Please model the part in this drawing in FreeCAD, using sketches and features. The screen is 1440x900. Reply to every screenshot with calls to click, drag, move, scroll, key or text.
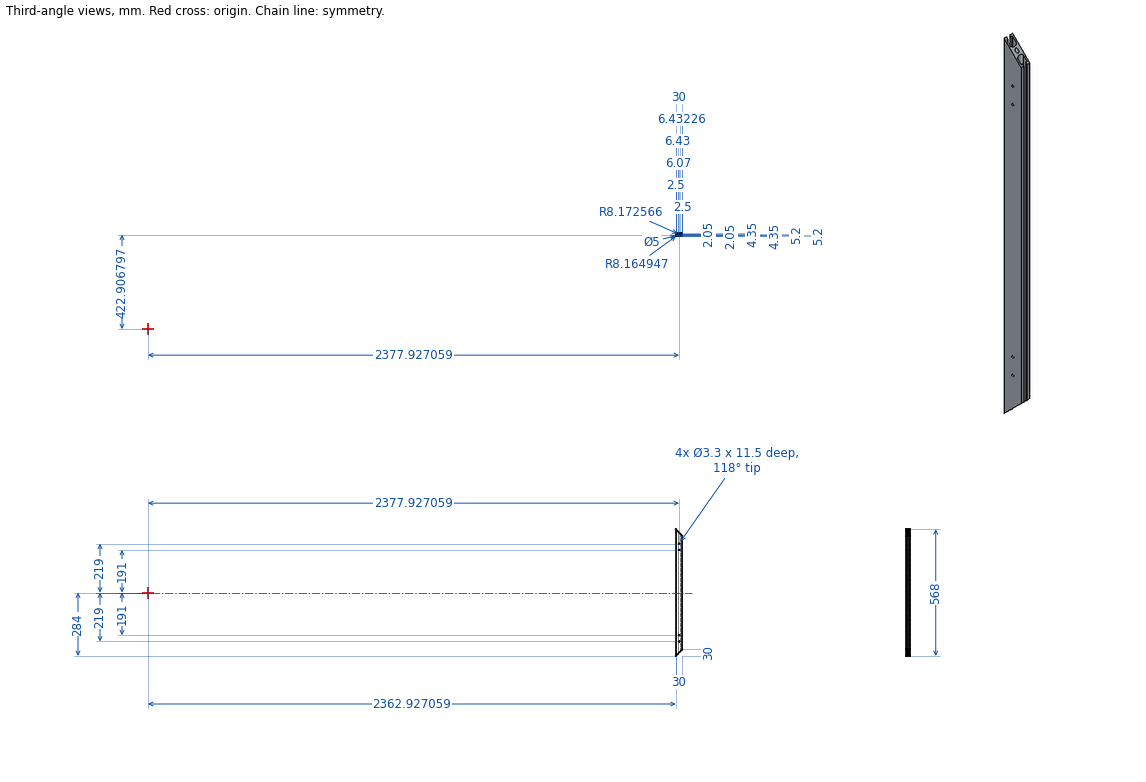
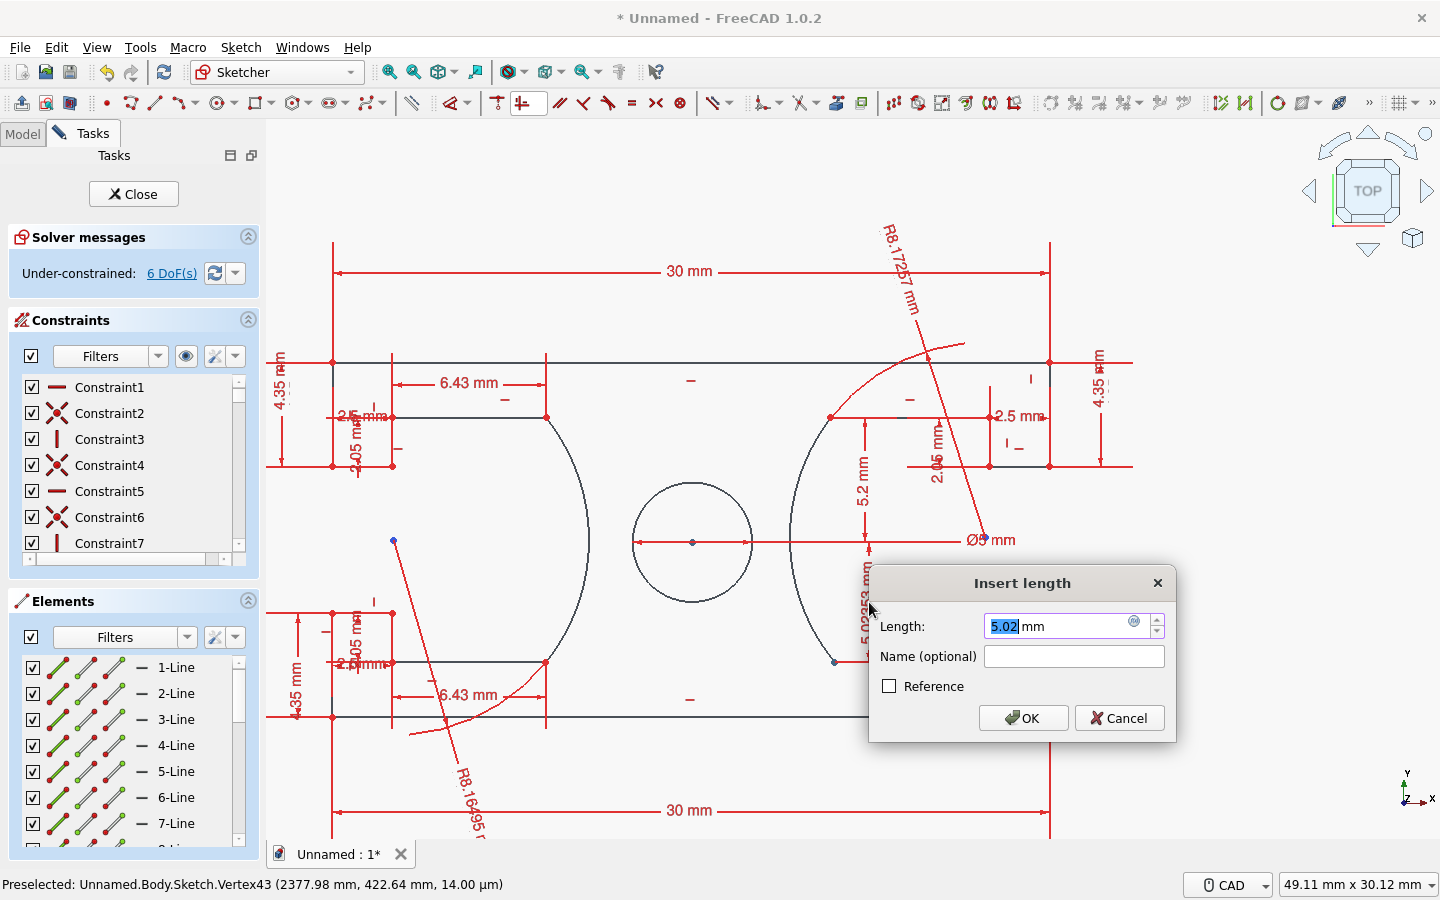
text(5.2)
key(Return)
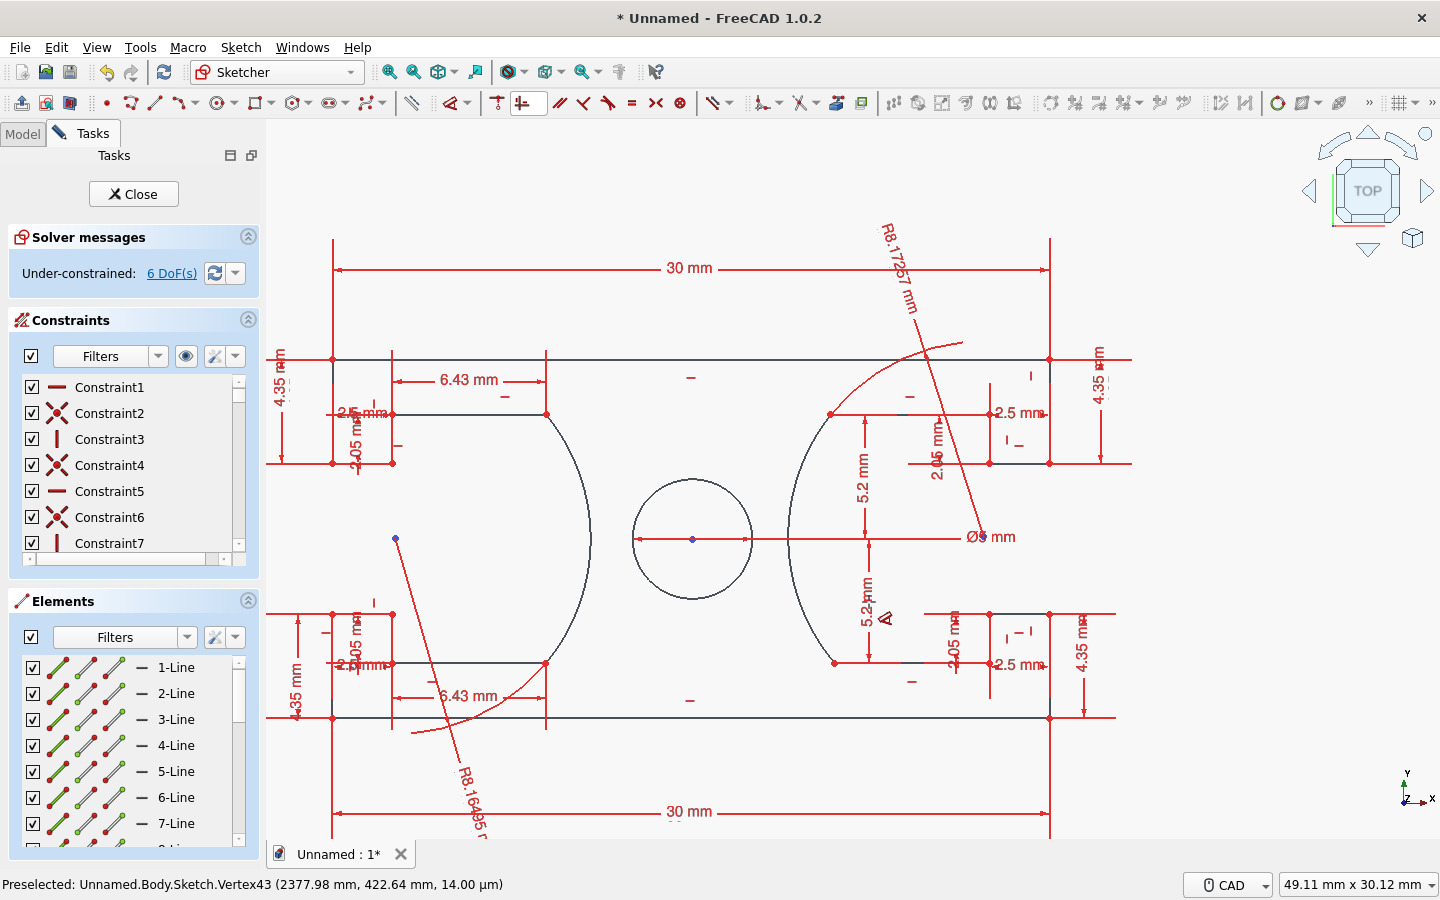
click(546, 415)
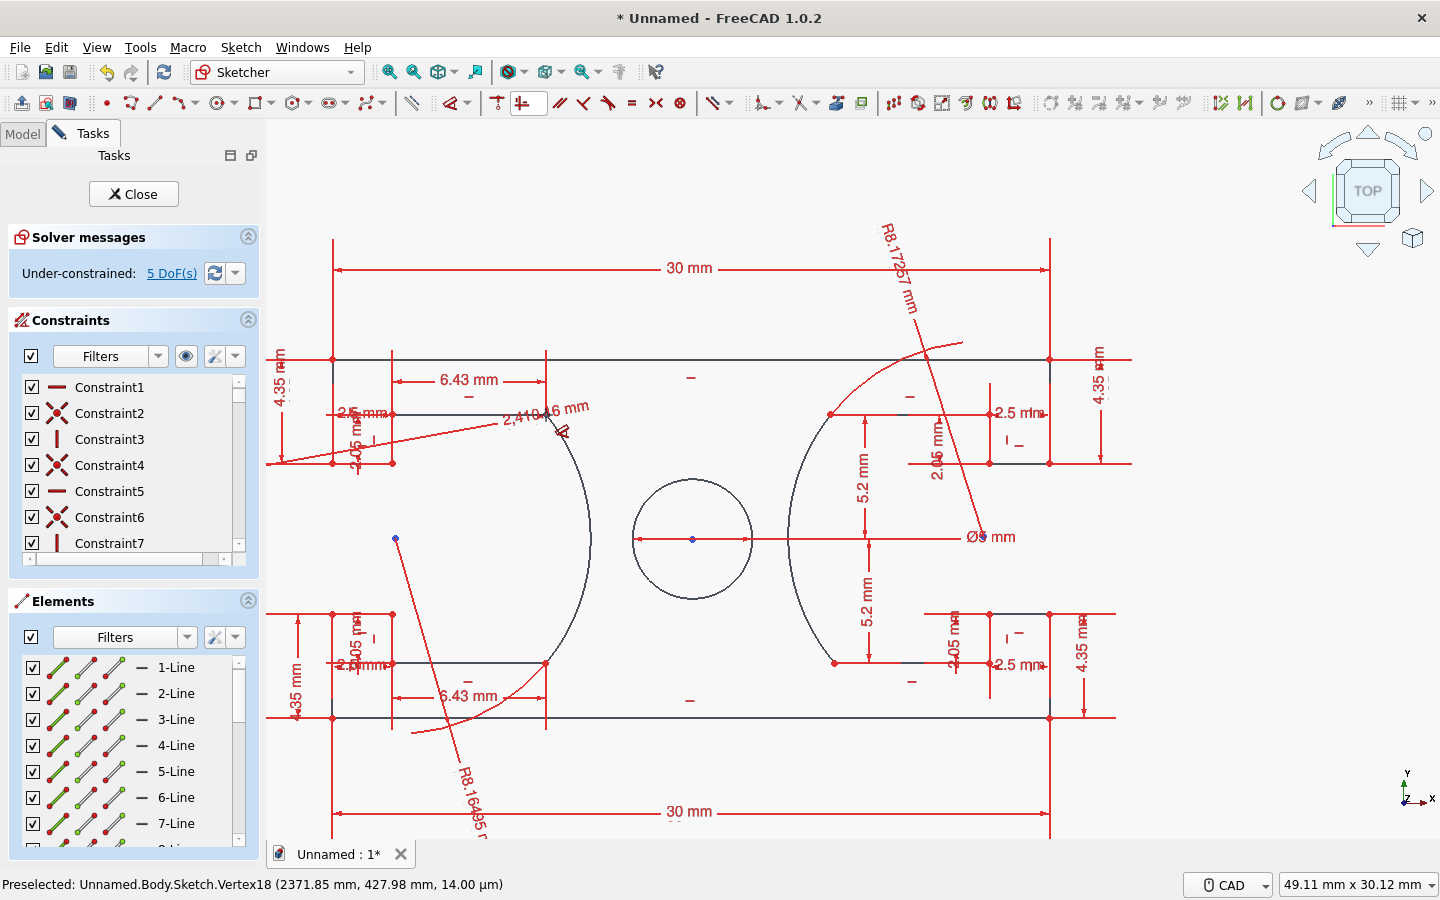
click(692, 539)
click(619, 381)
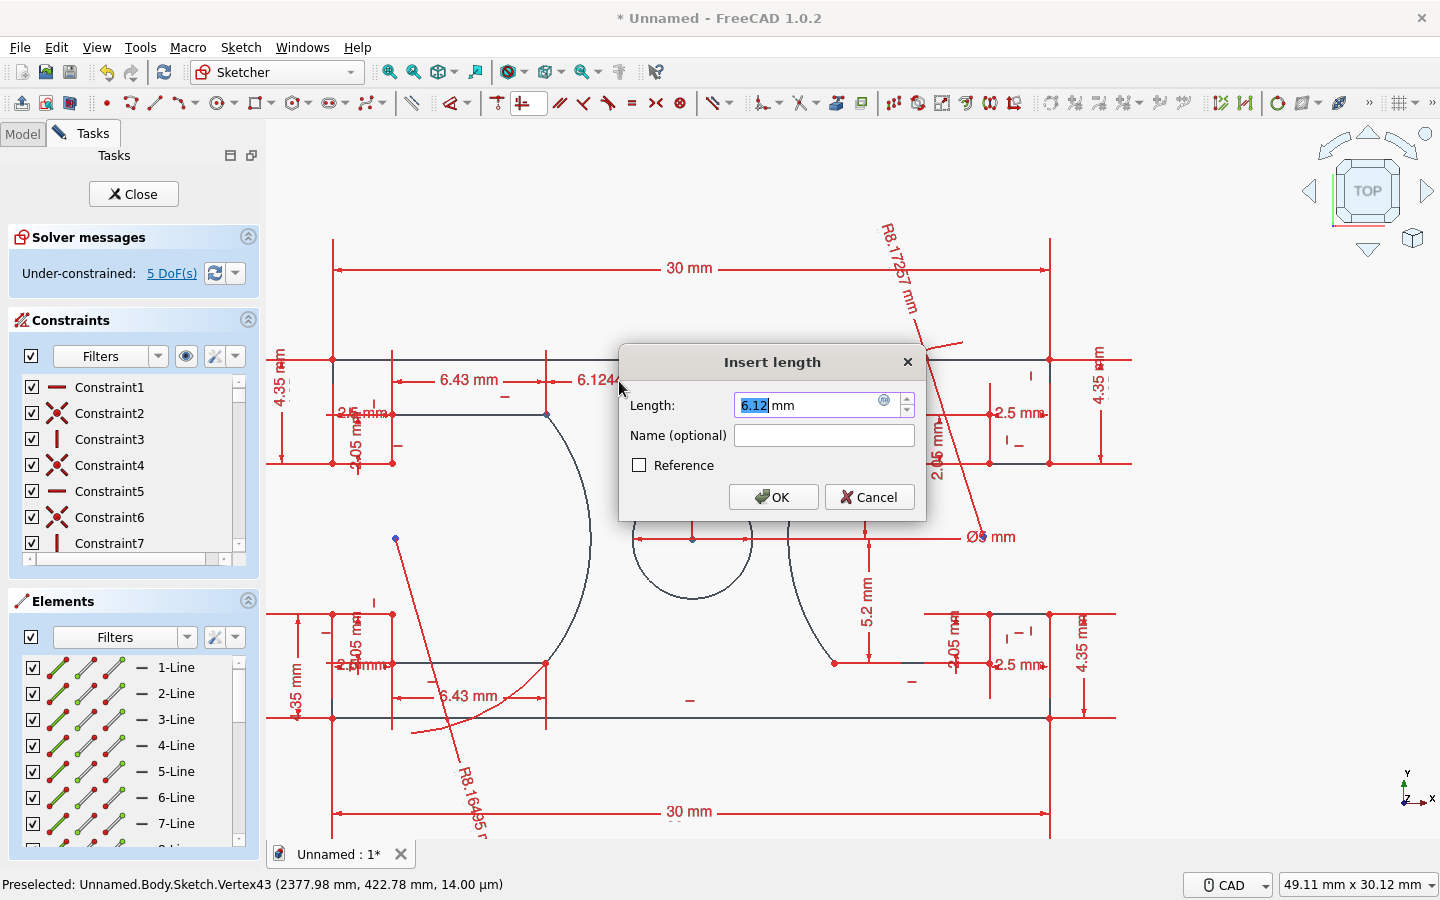
text(6.07)
key(Return)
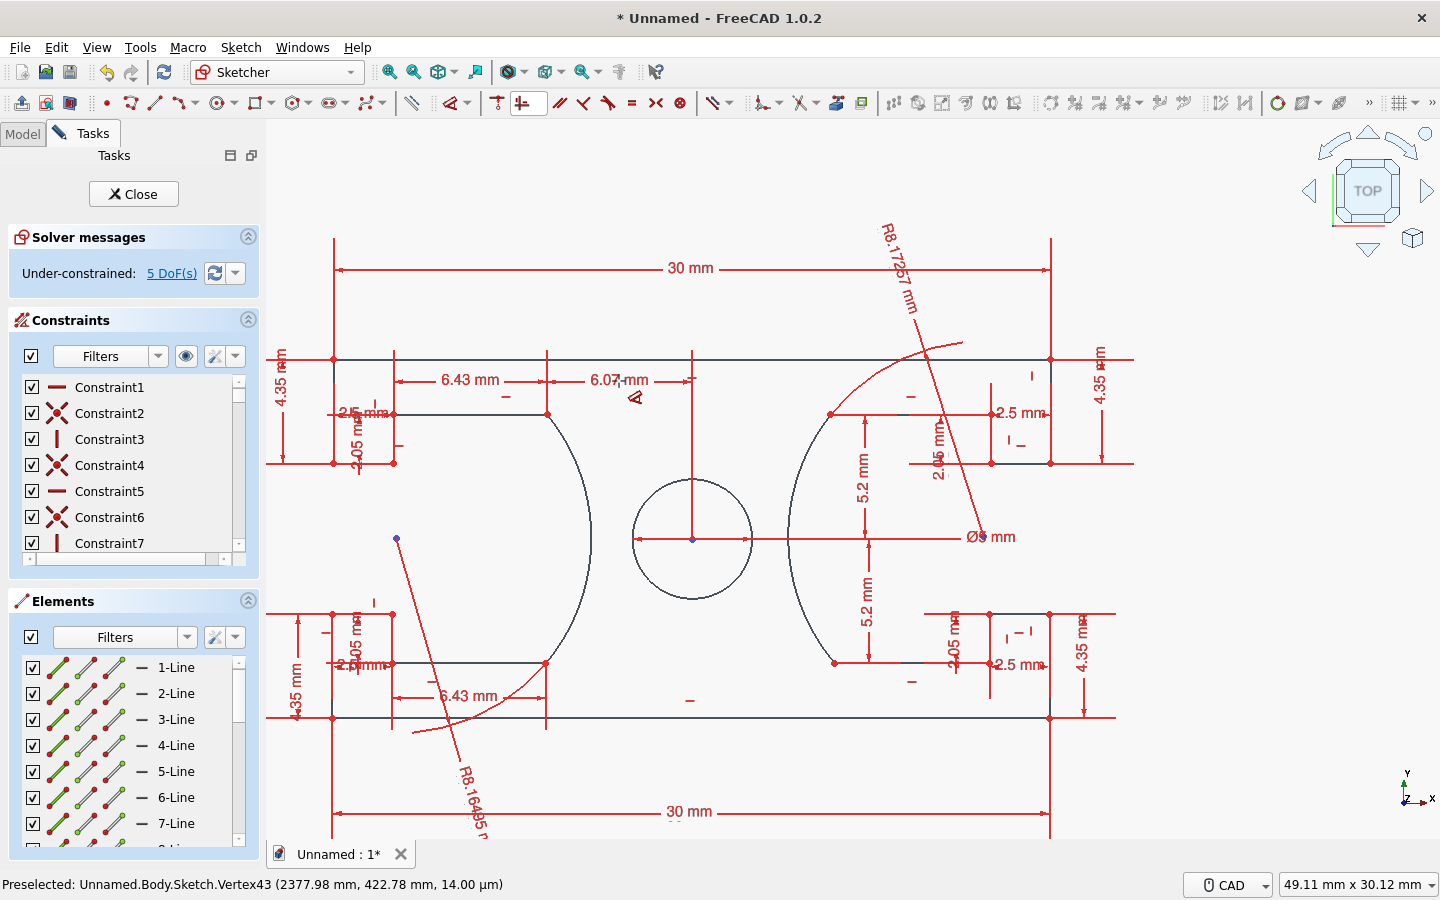
click(546, 663)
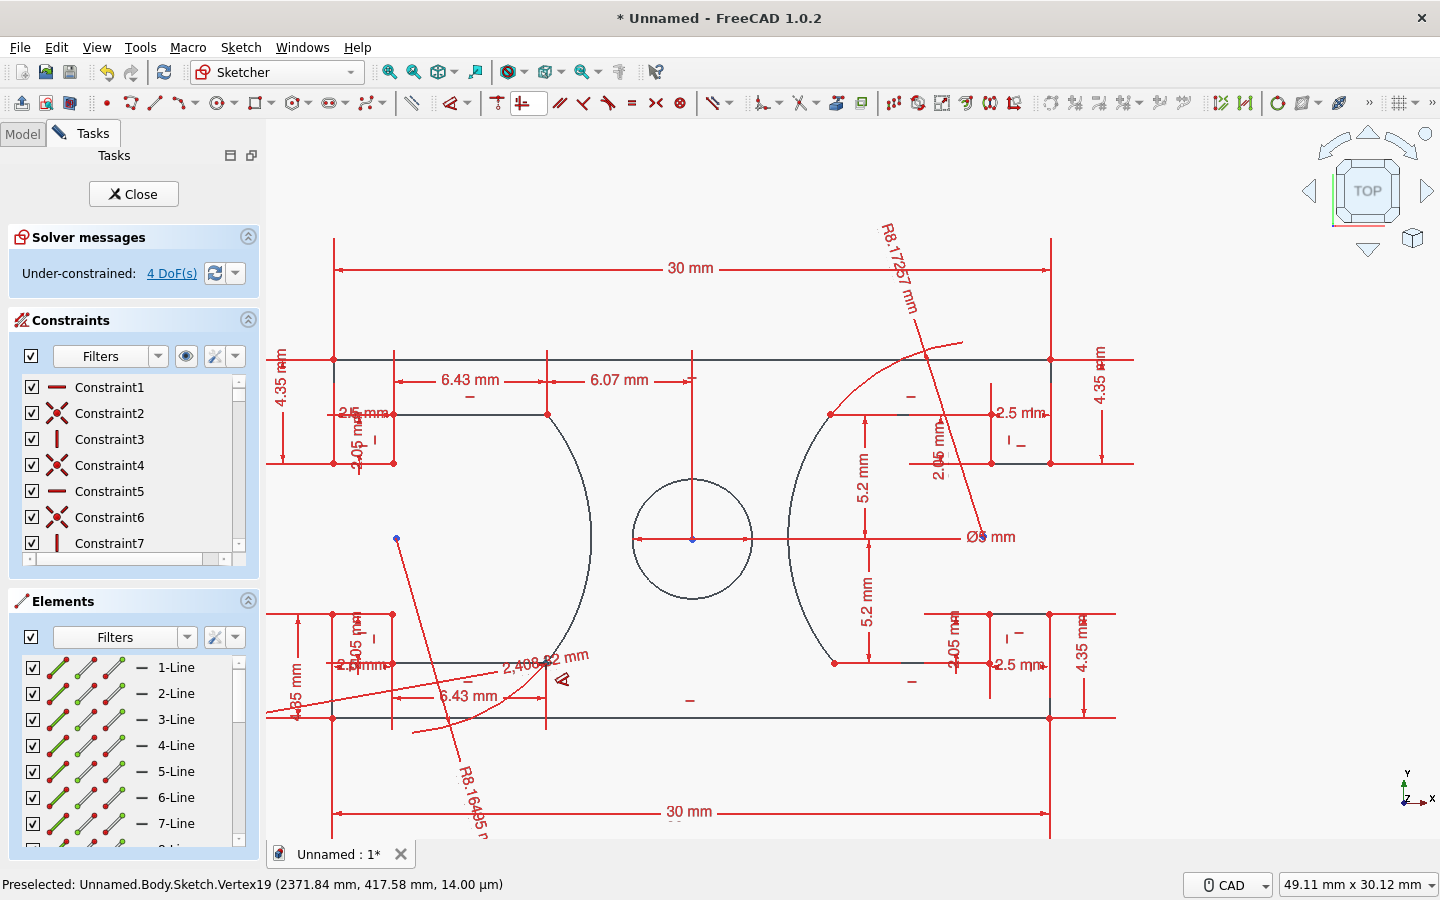
click(692, 539)
click(619, 697)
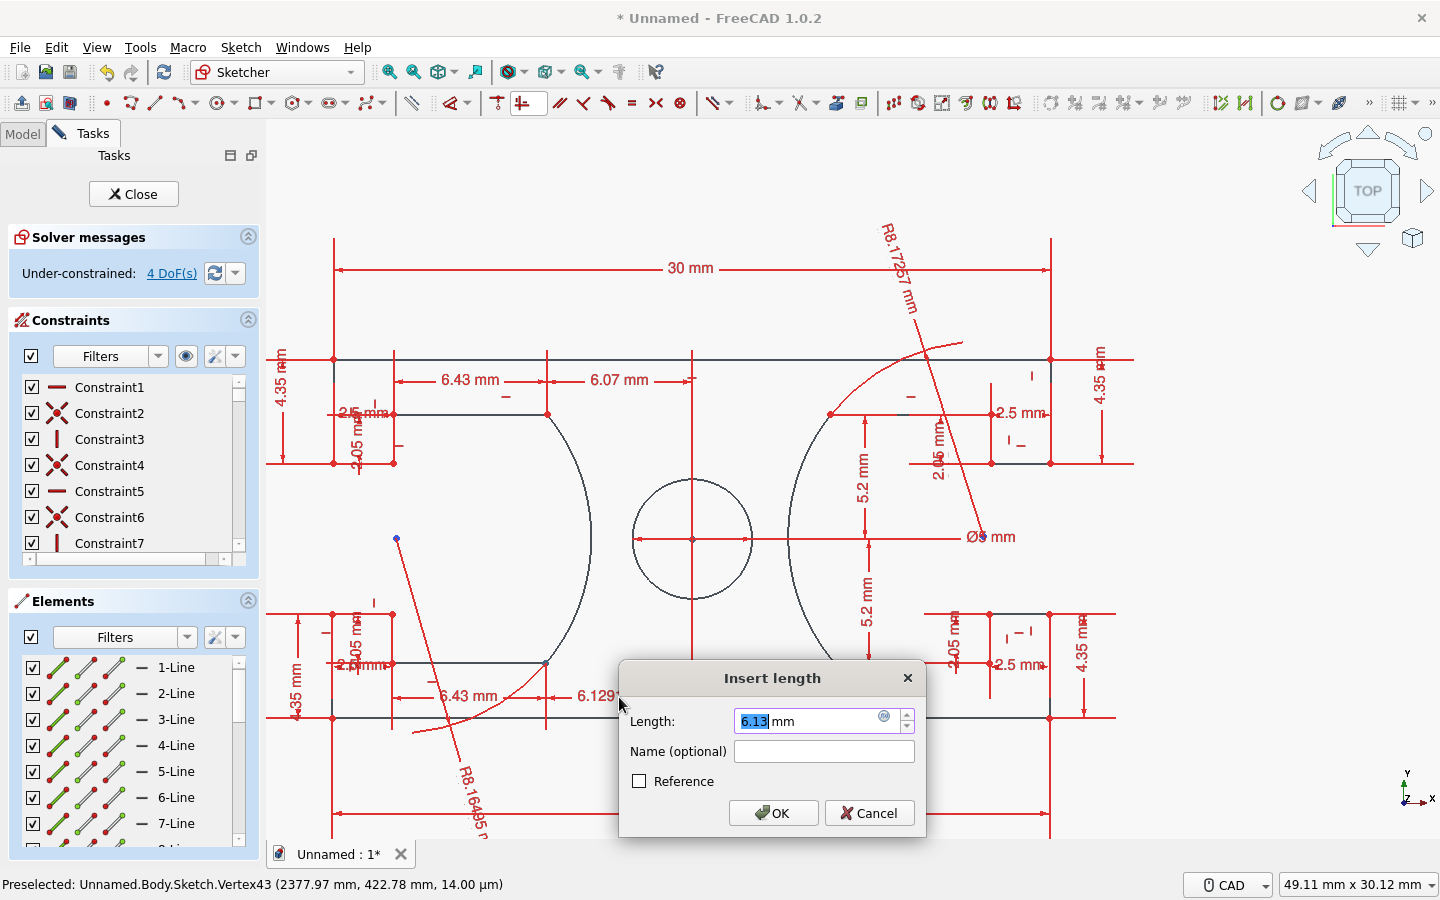
text(6.07)
key(Return)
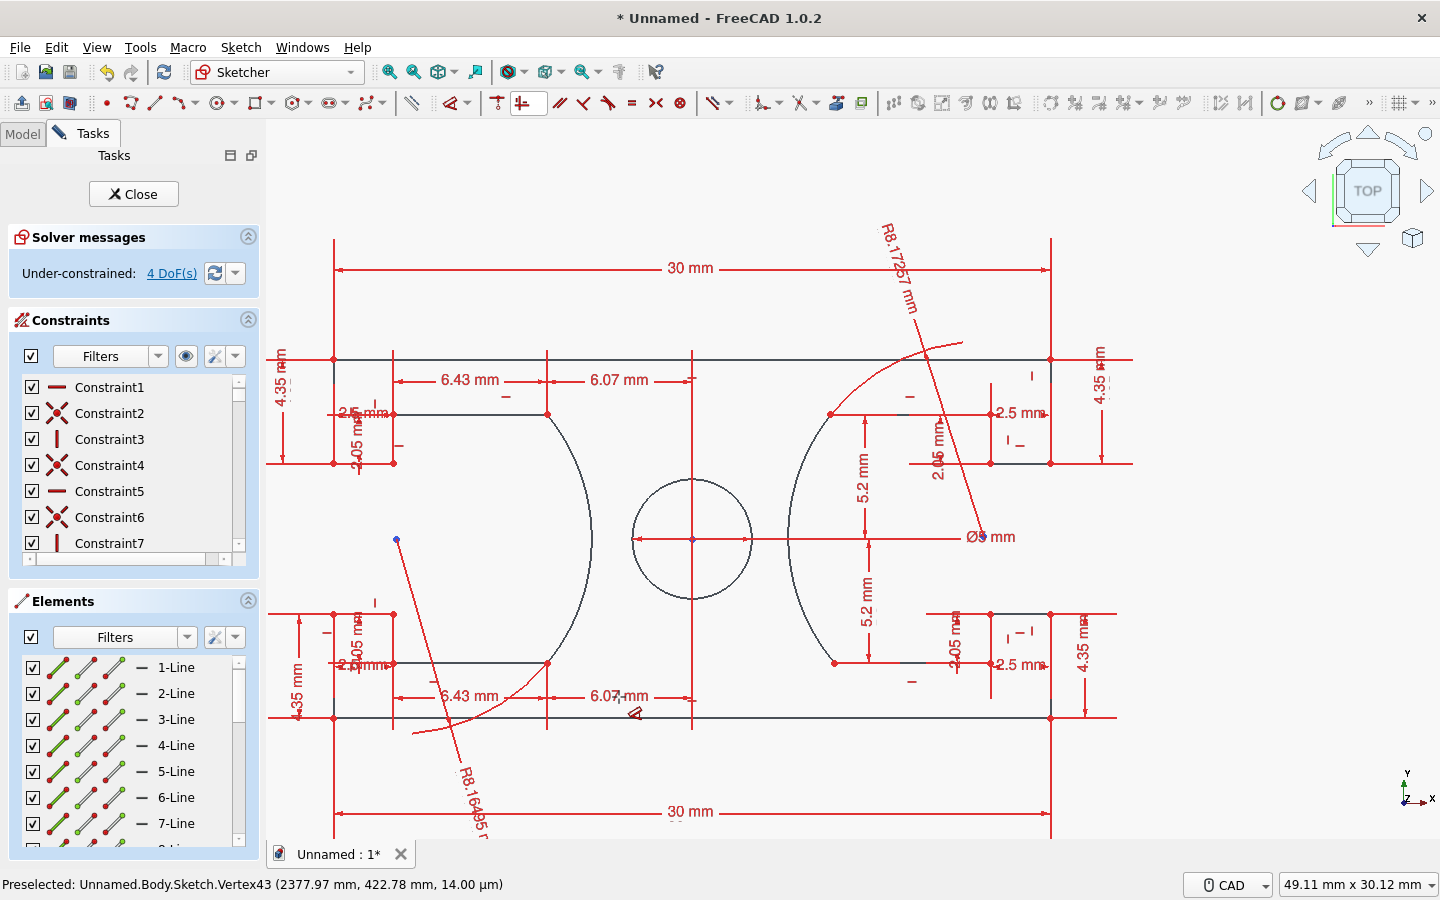
click(879, 415)
click(911, 381)